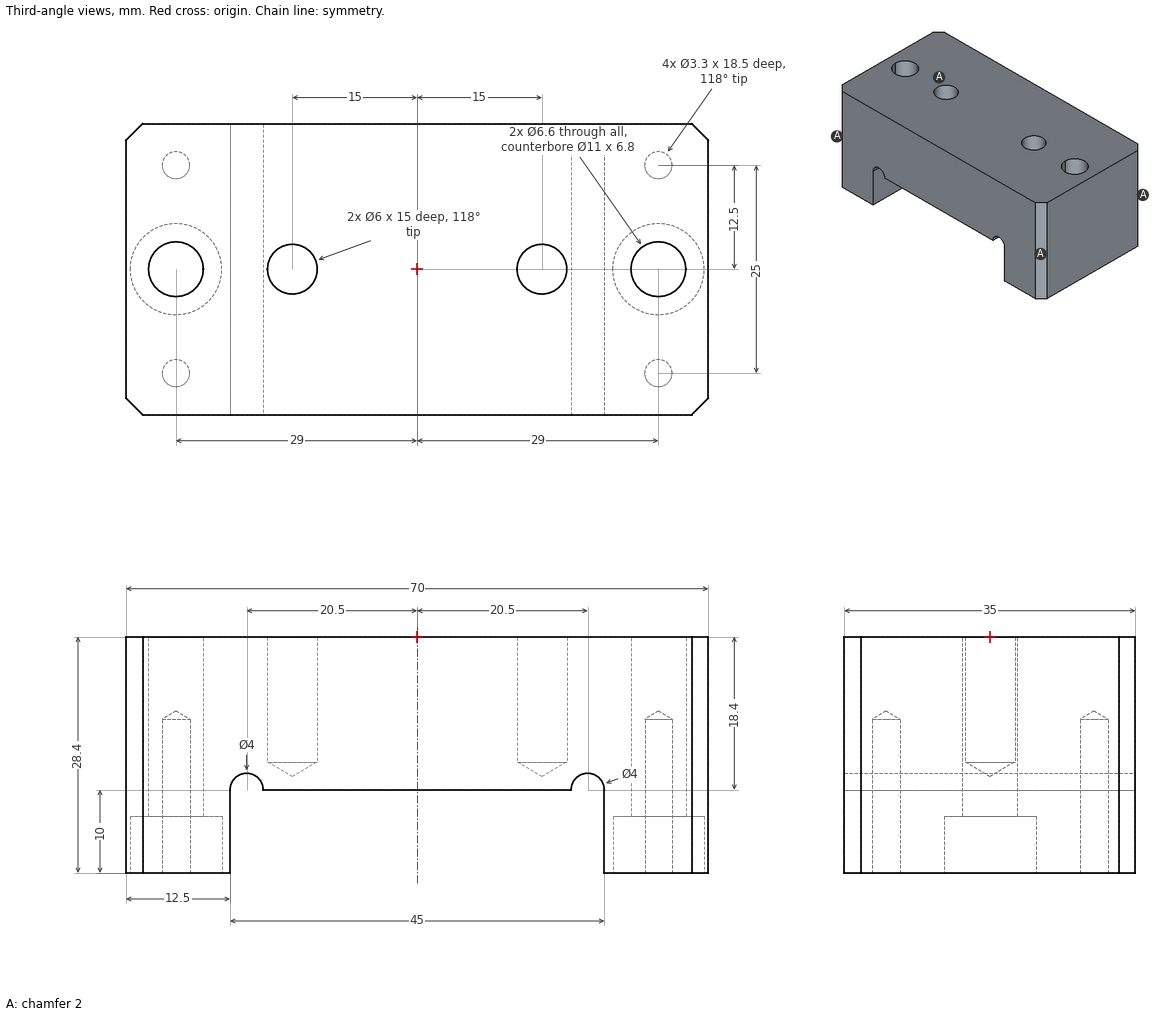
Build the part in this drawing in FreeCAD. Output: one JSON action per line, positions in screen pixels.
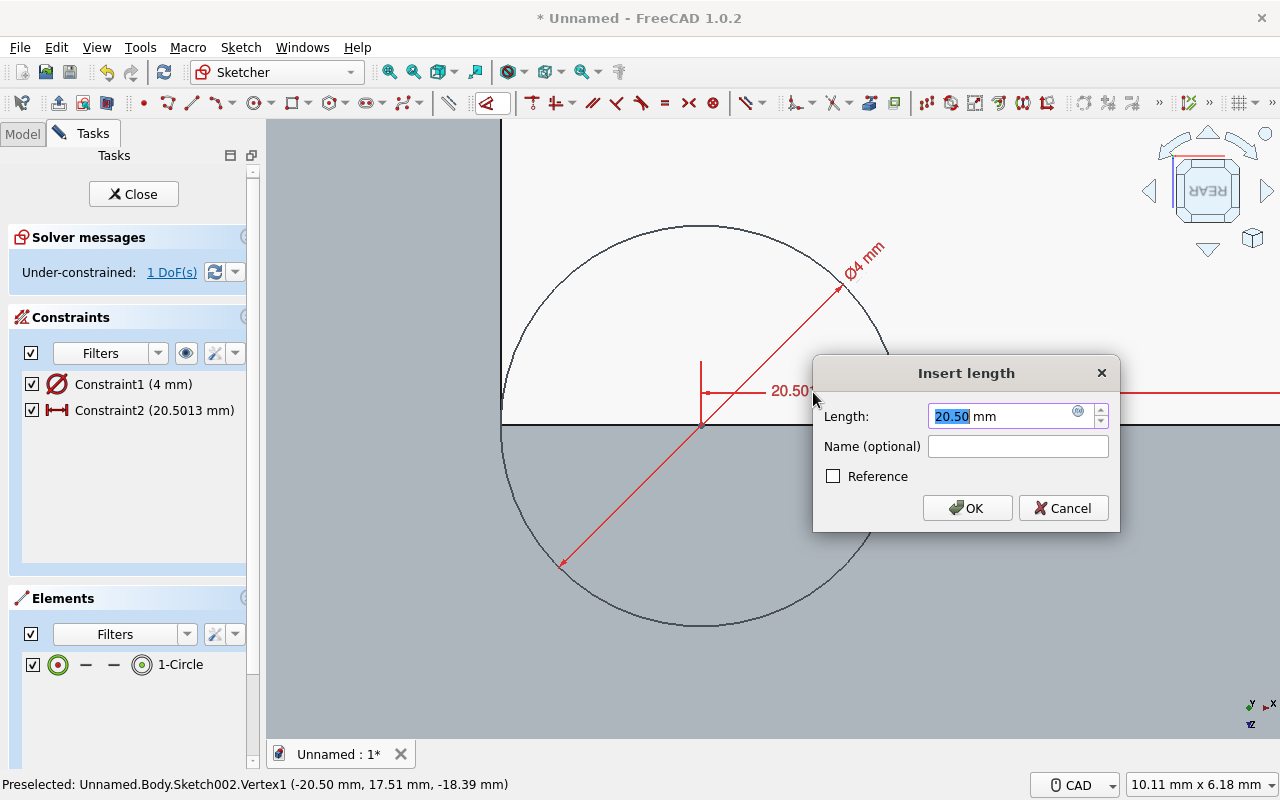
{"action": "type", "text": "20.5"}
{"action": "key", "text": "Return"}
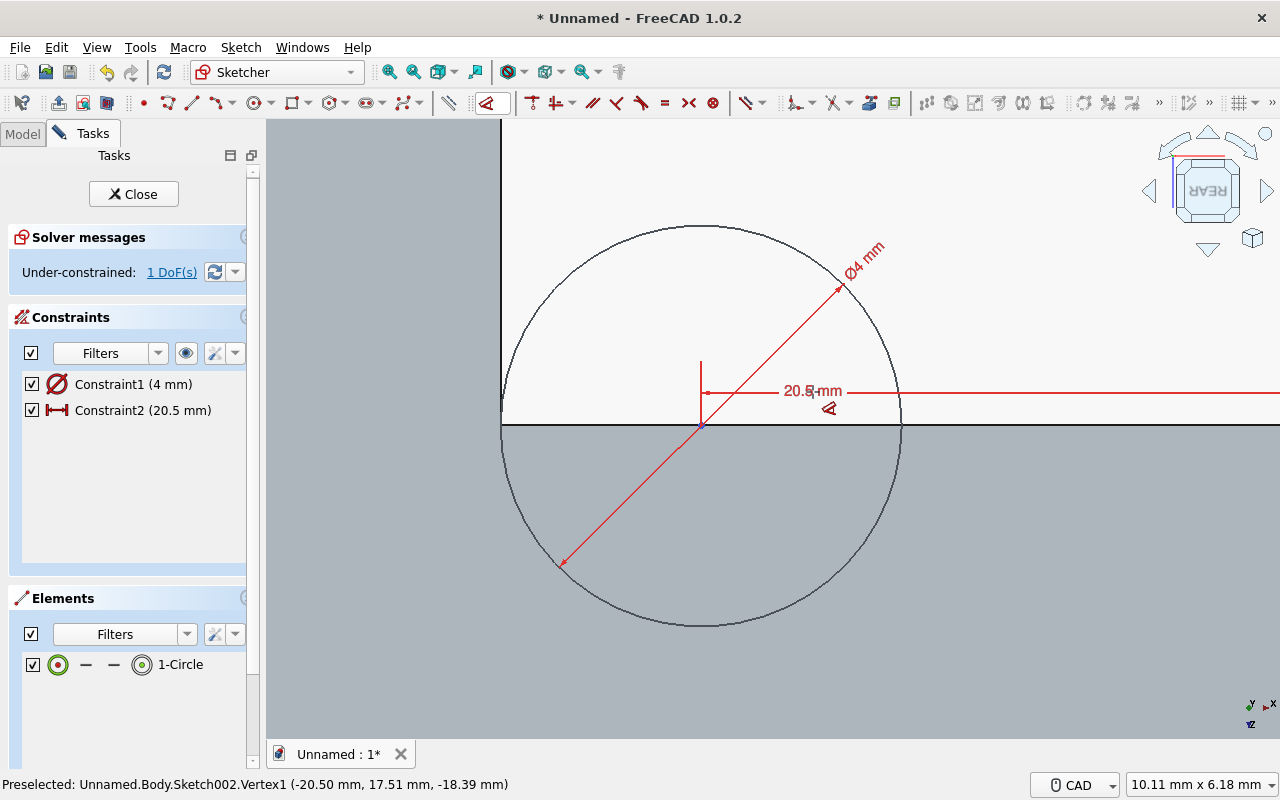
{"action": "left_click", "coordinate": [701, 426]}
{"action": "left_click", "coordinate": [667, 569]}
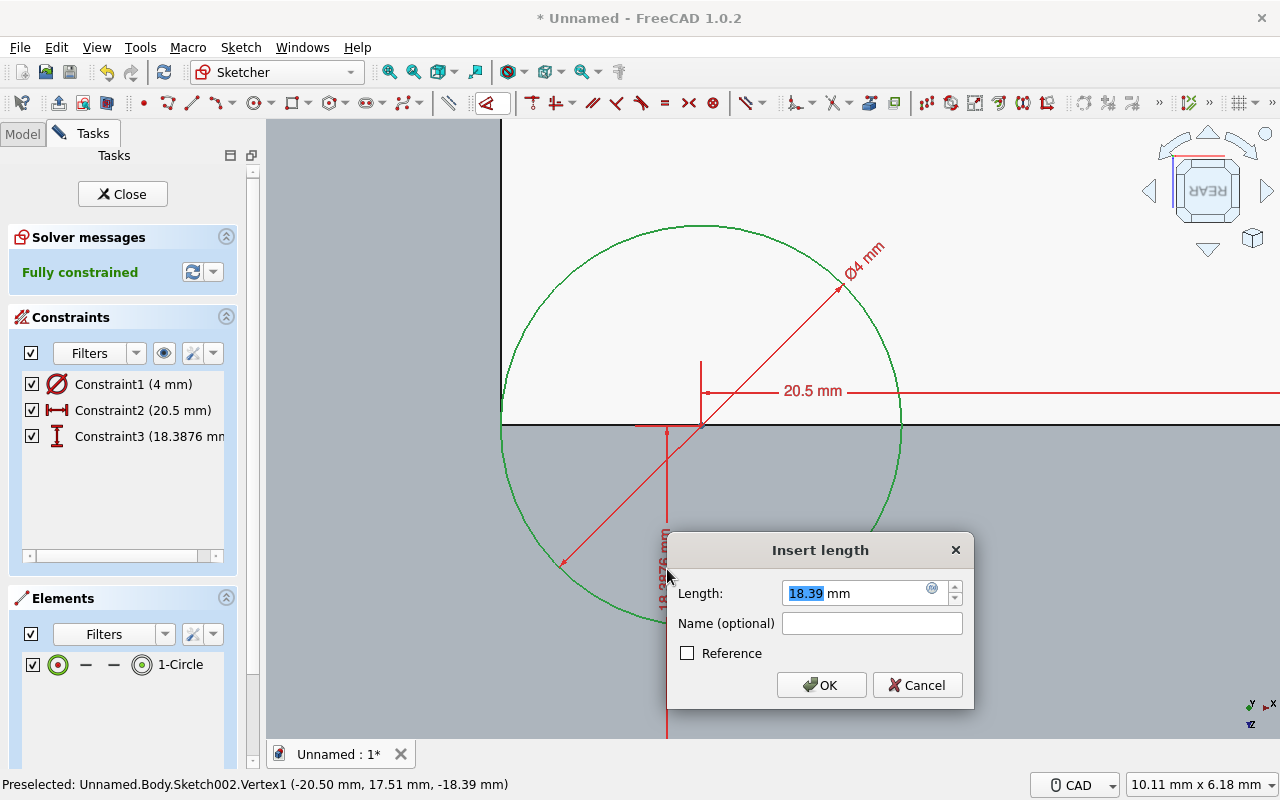
{"action": "type", "text": "18.4"}
{"action": "key", "text": "Return"}
{"action": "key", "text": "Escape"}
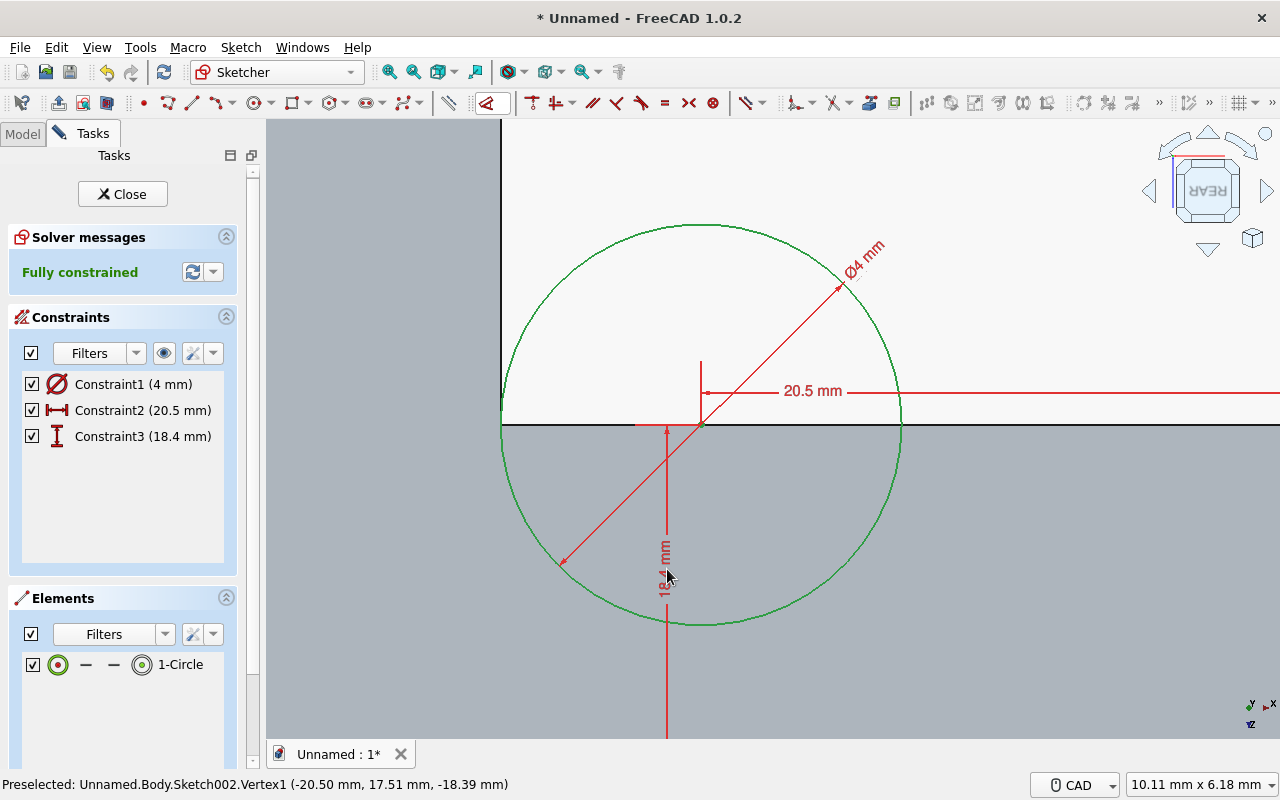
{"action": "left_click", "coordinate": [123, 194]}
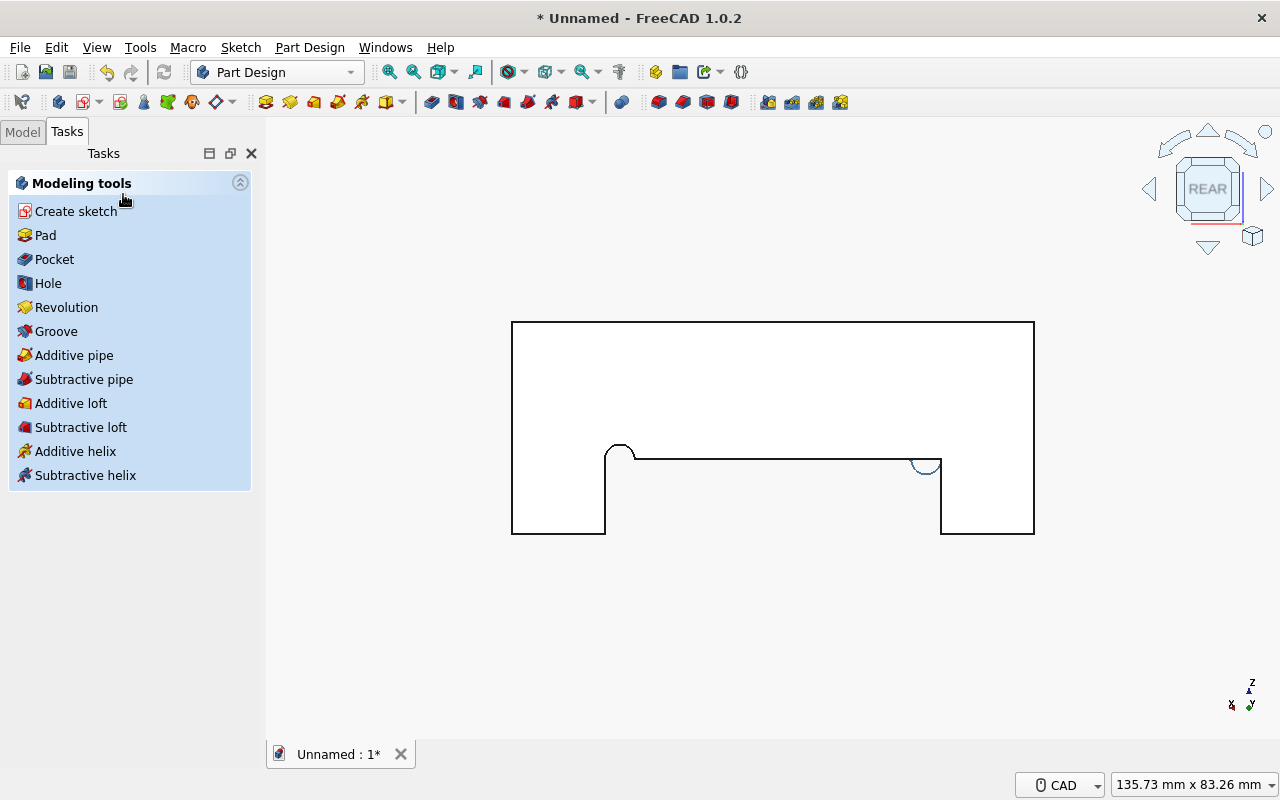
{"action": "left_click", "coordinate": [432, 102]}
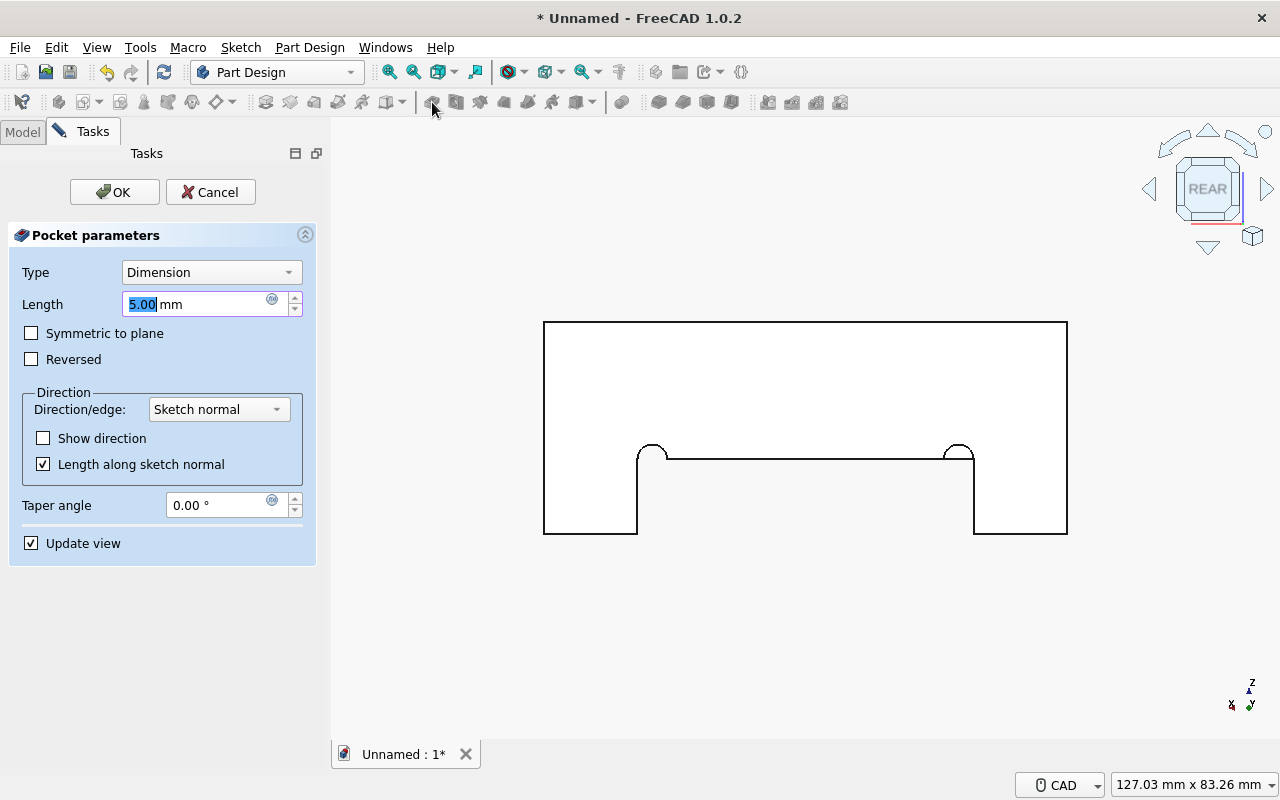
{"action": "left_click", "coordinate": [212, 272]}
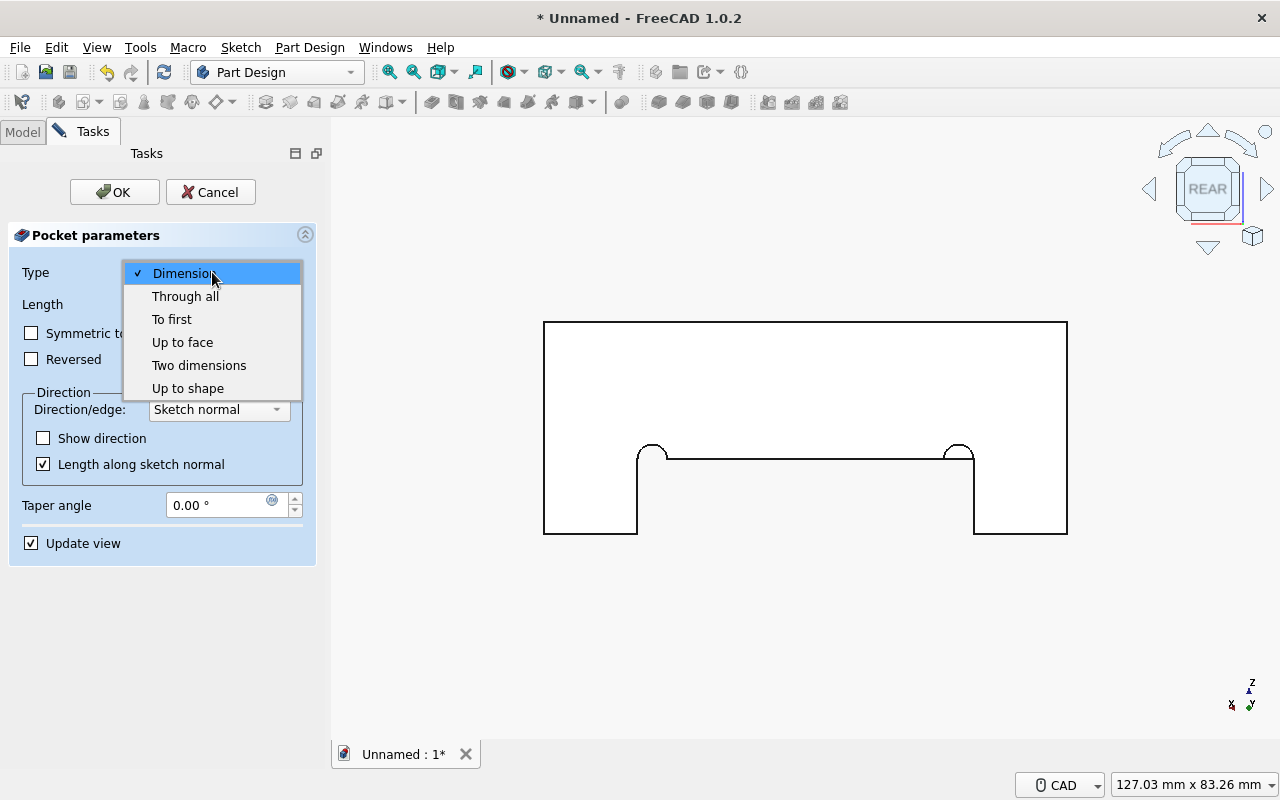
{"action": "left_click", "coordinate": [212, 320]}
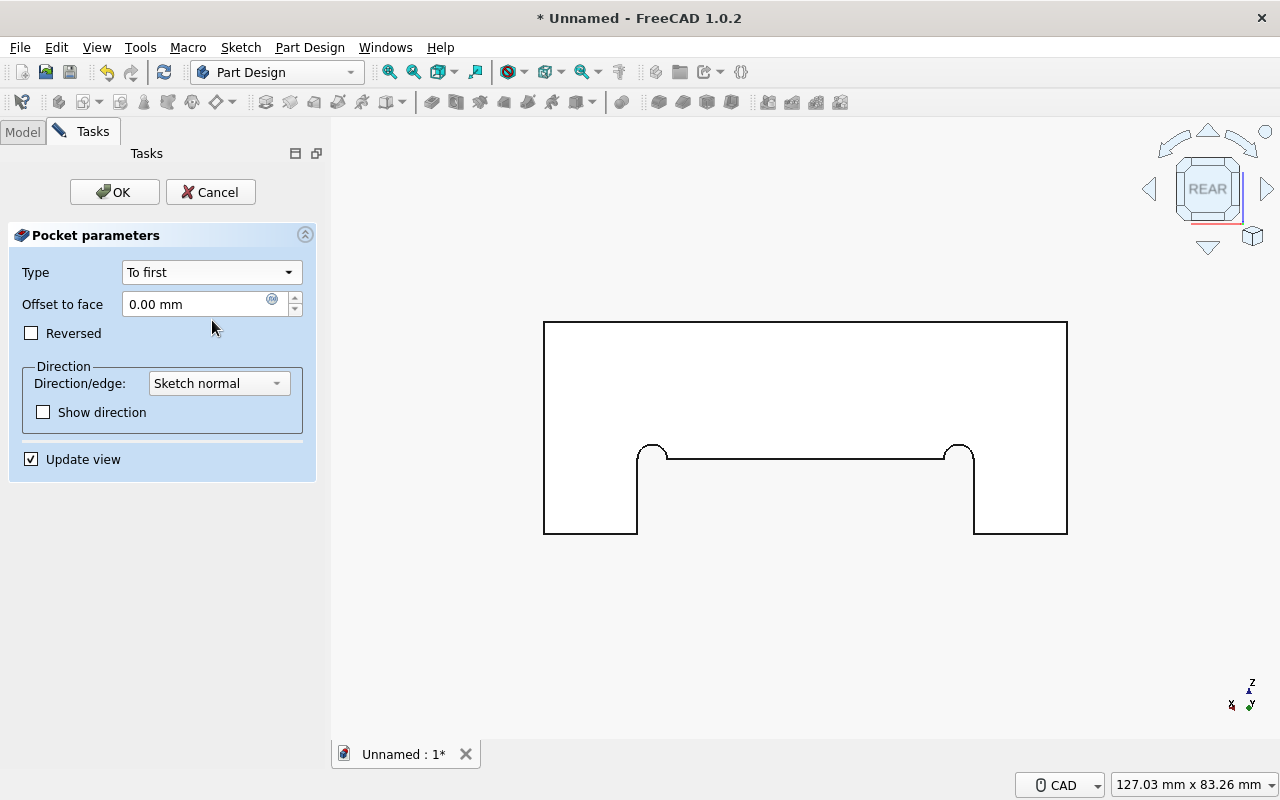
{"action": "left_click", "coordinate": [115, 192]}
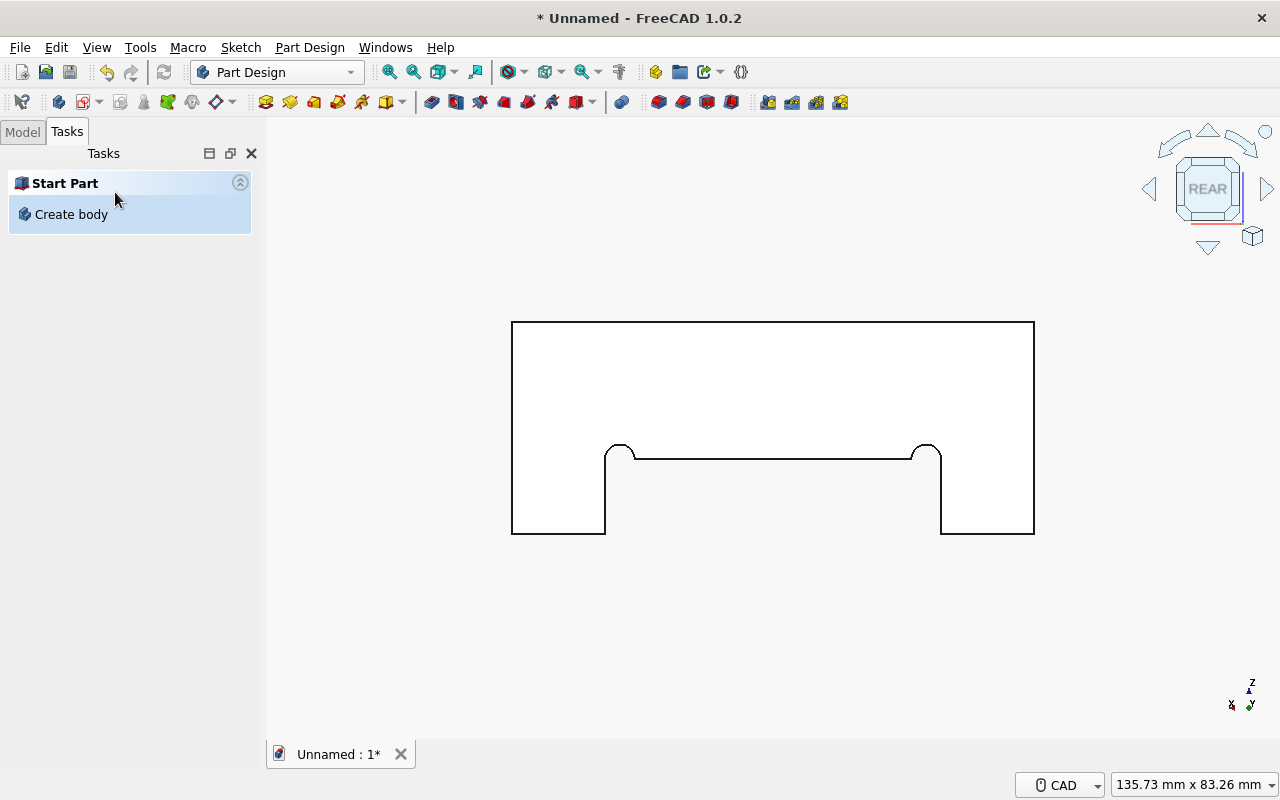
{"action": "left_click", "coordinate": [1034, 427]}